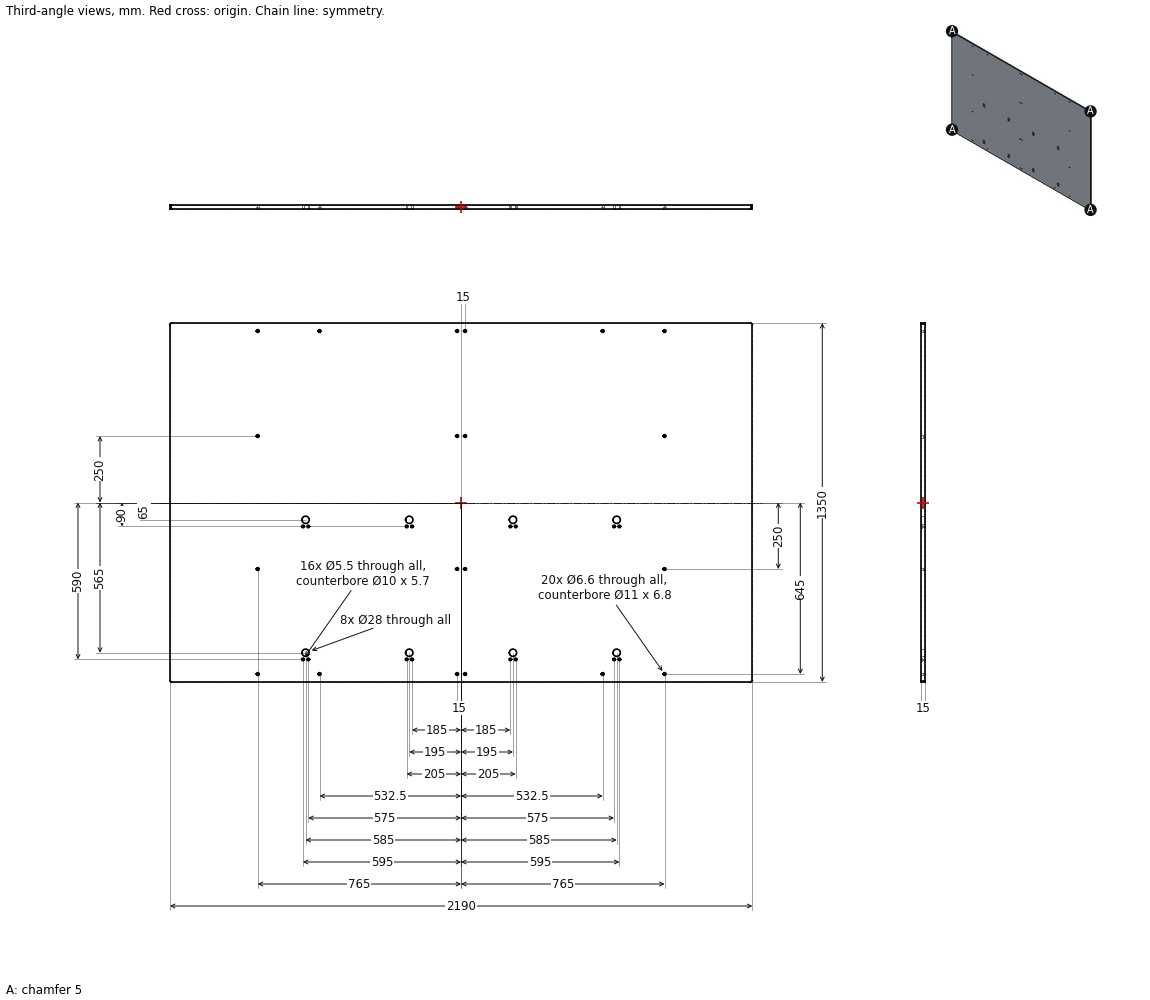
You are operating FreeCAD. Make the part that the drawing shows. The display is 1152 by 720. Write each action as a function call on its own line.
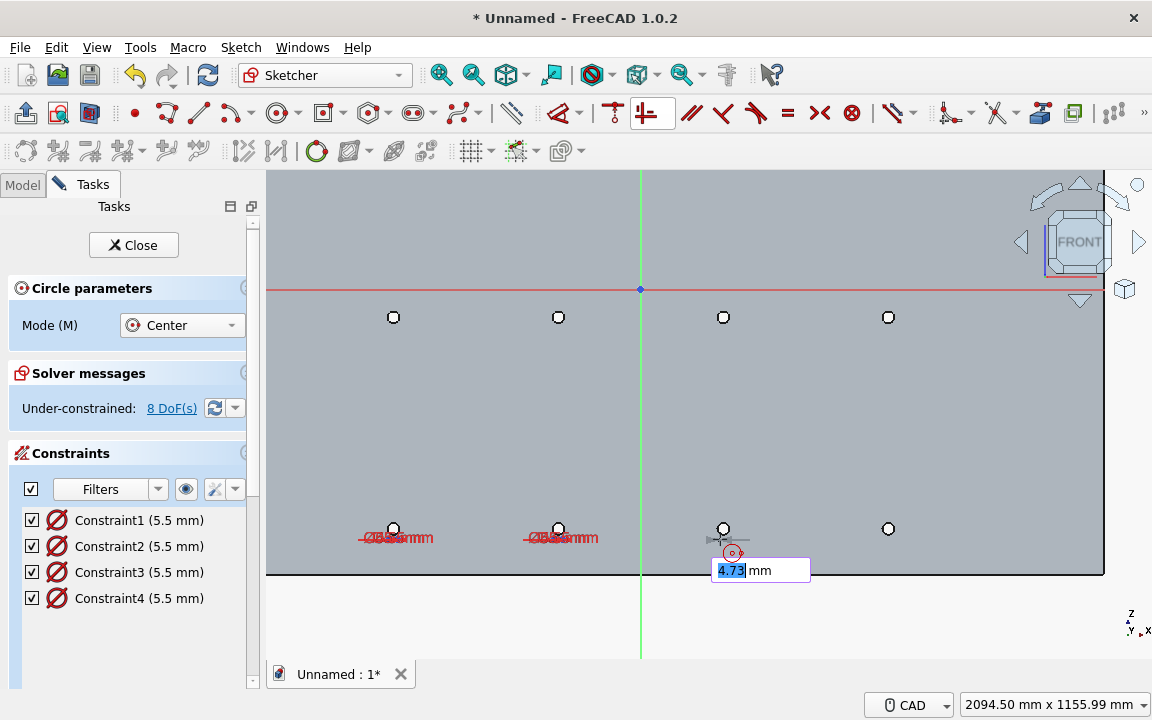
text(5.5)
key(Return)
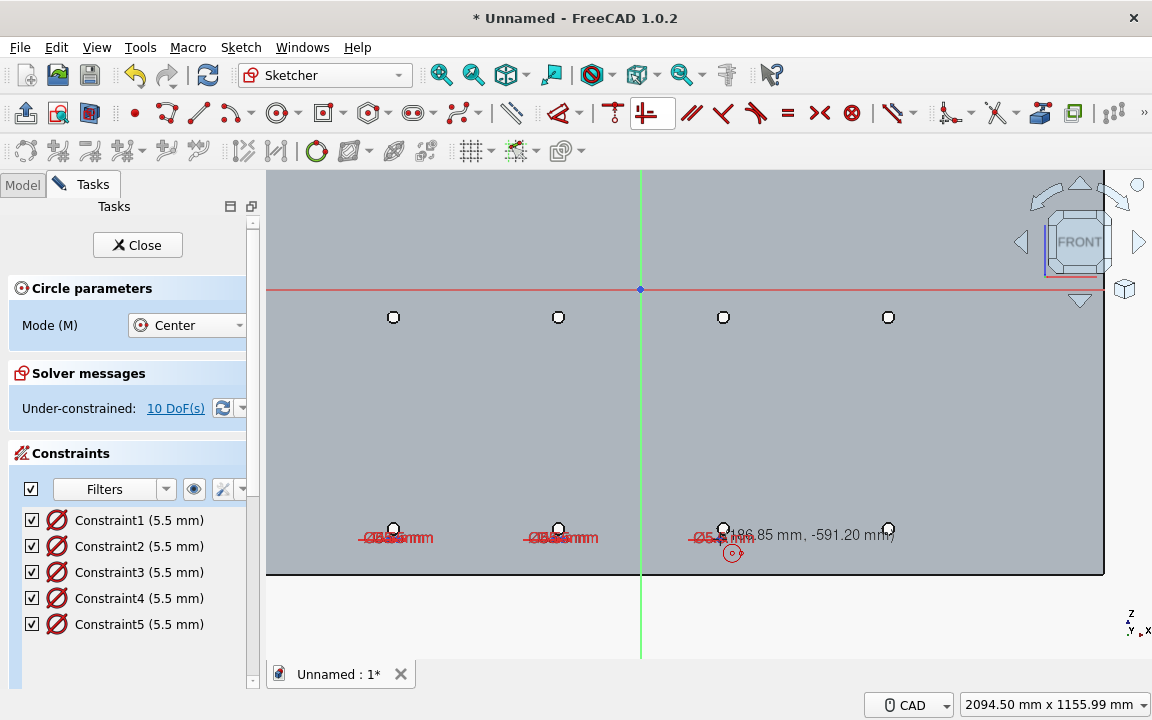
scroll(728, 539, up, 15)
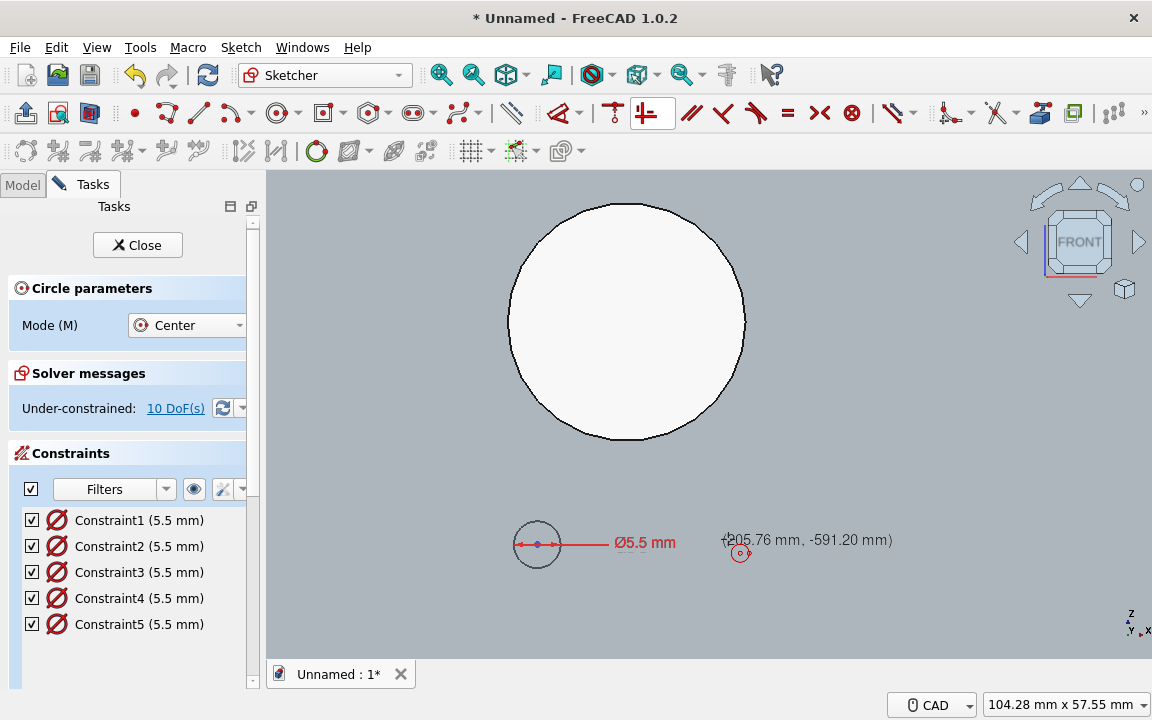
scroll(728, 539, down, 15)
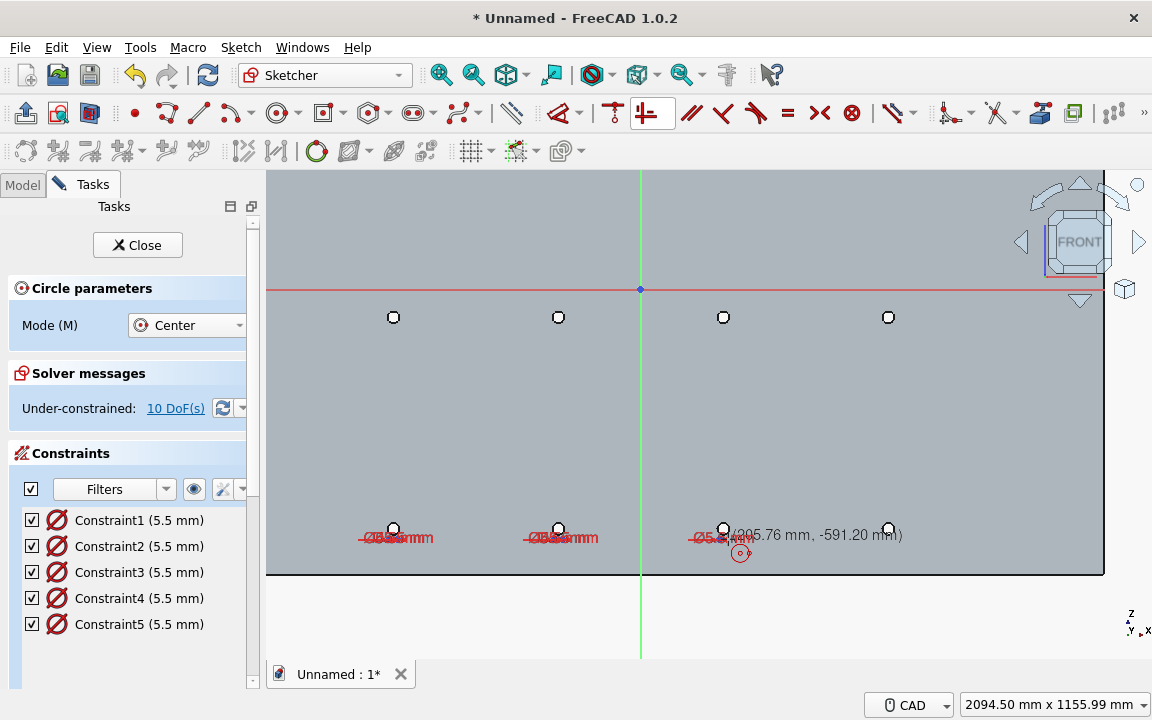
scroll(728, 539, up, 4)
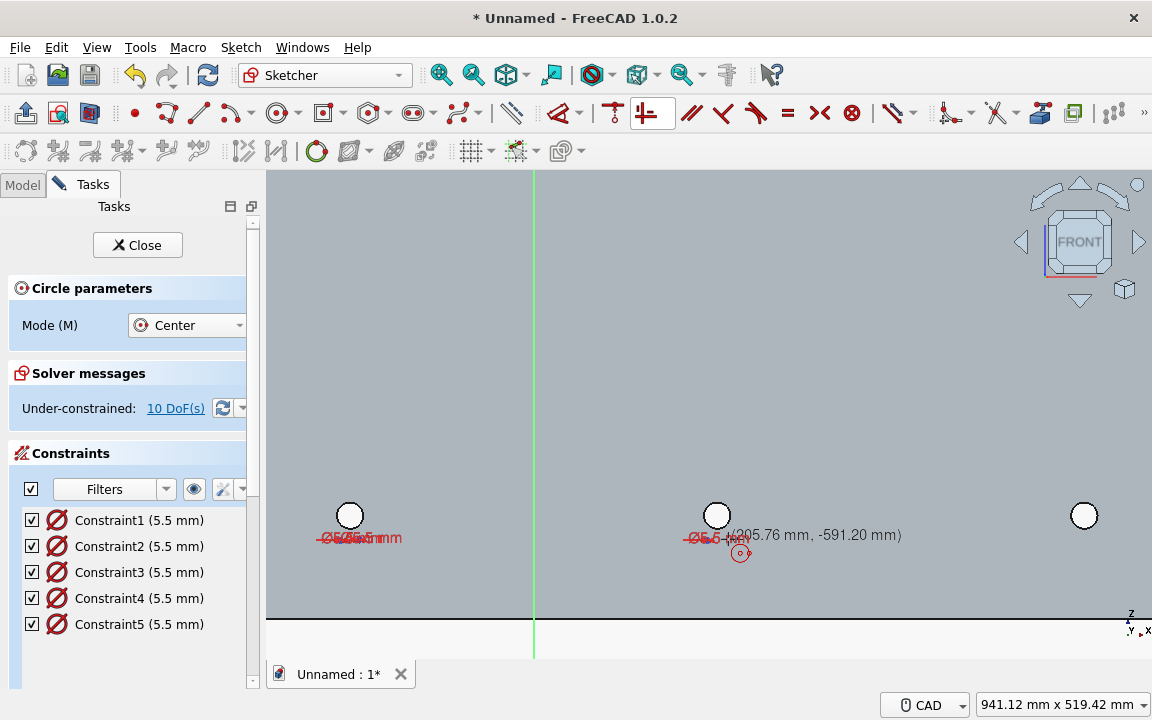
click(727, 539)
move(728, 537)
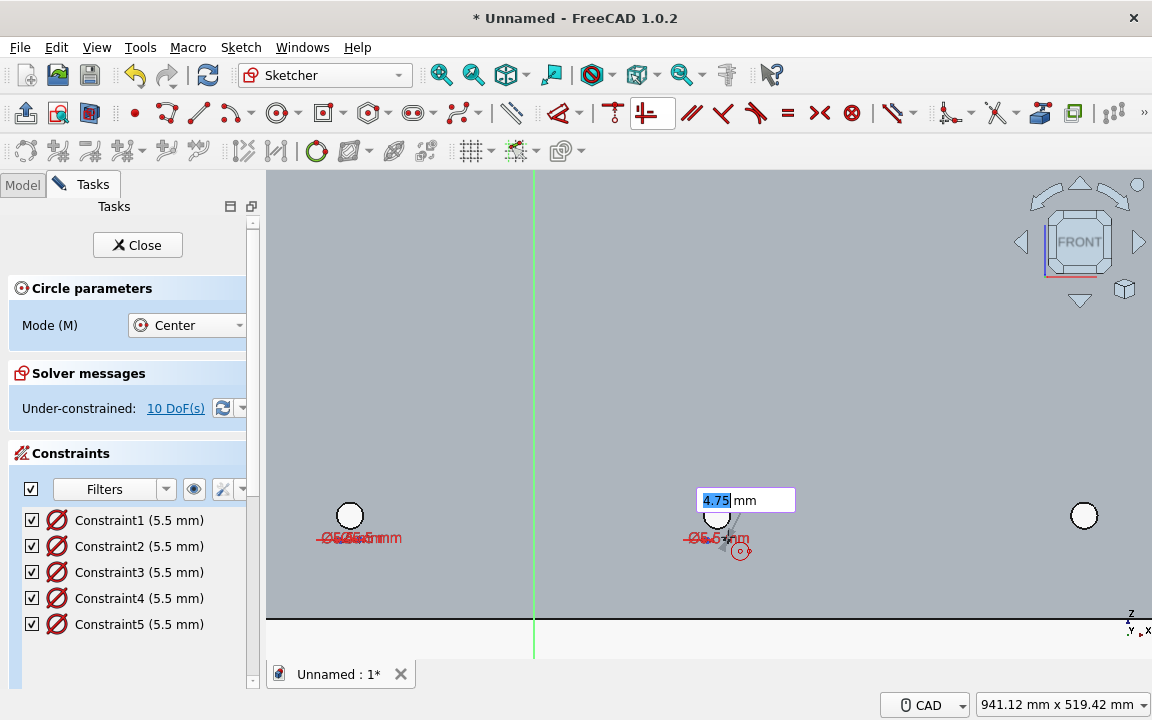
text(5.5)
key(Return)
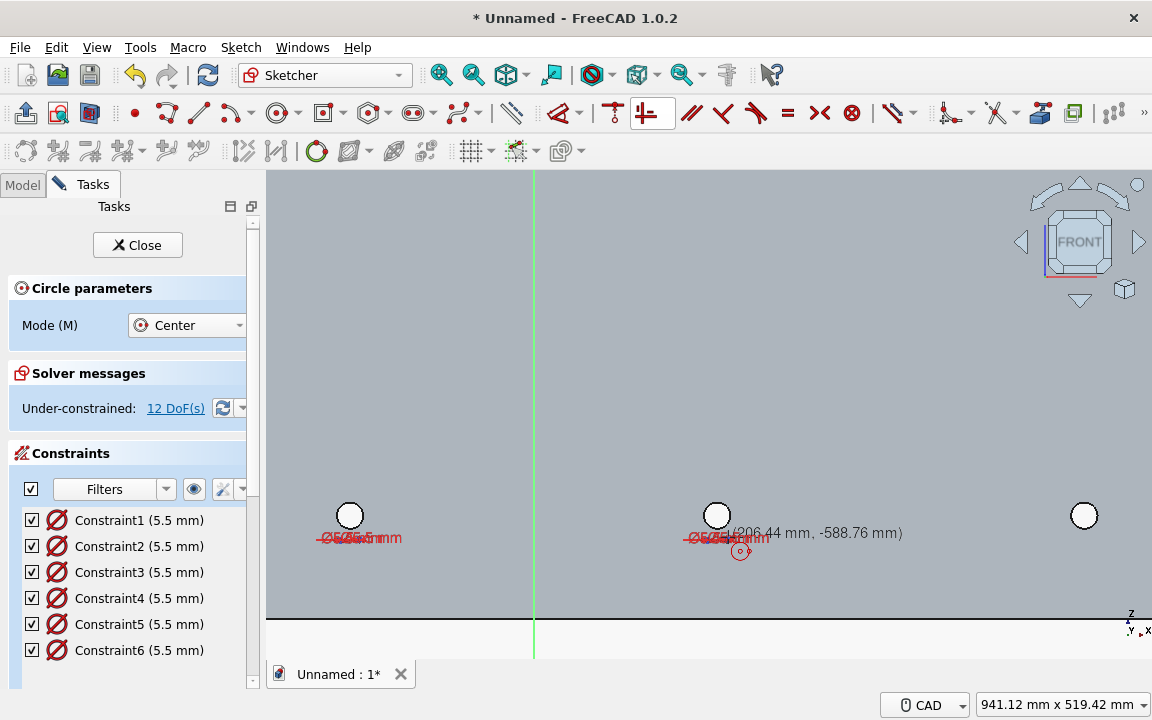
scroll(728, 538, down, 4)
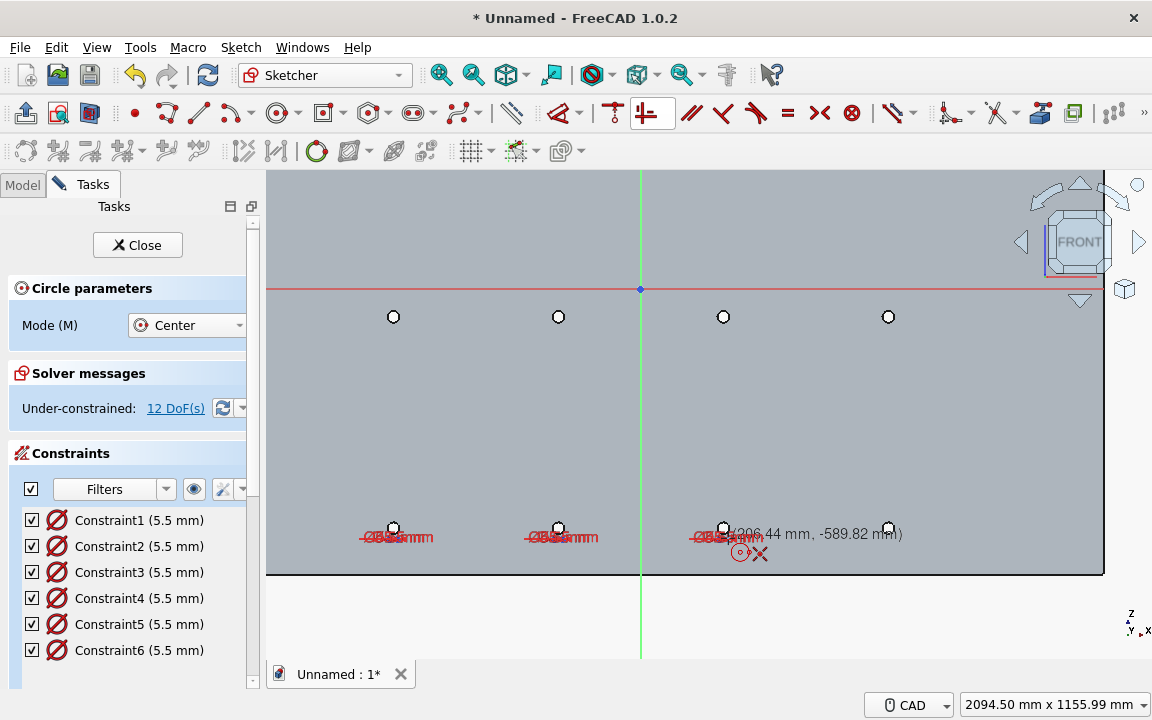
scroll(884, 539, up, 15)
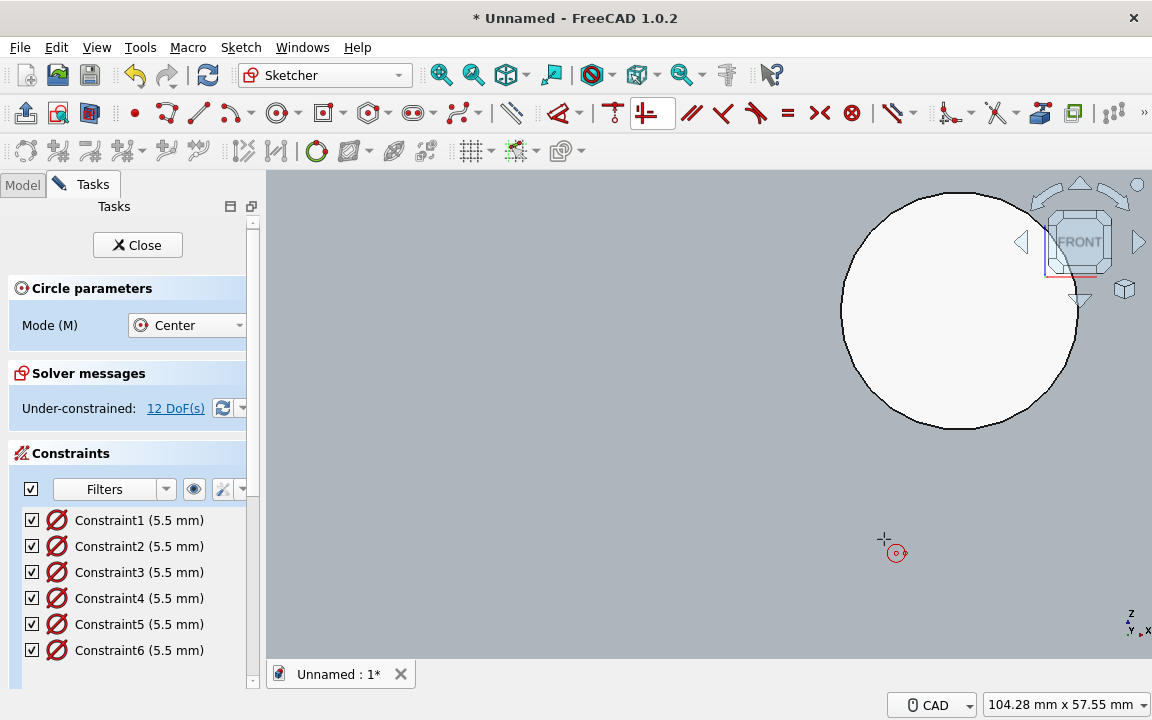
scroll(884, 540, down, 15)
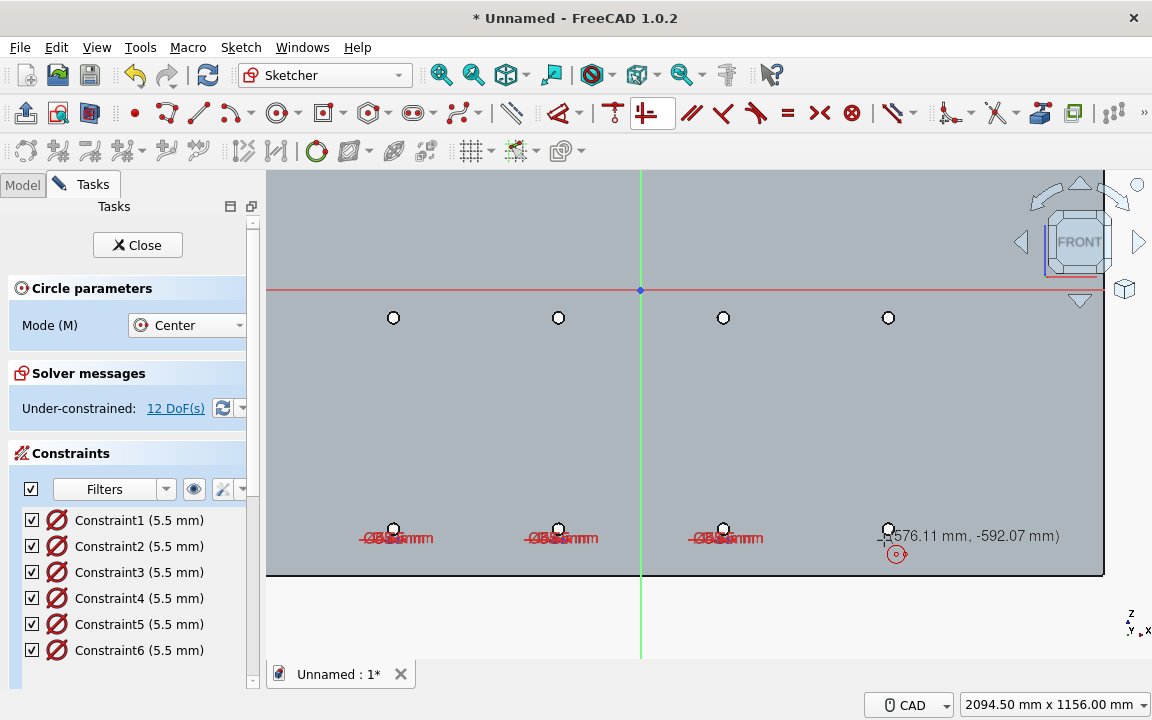
click(884, 540)
move(885, 539)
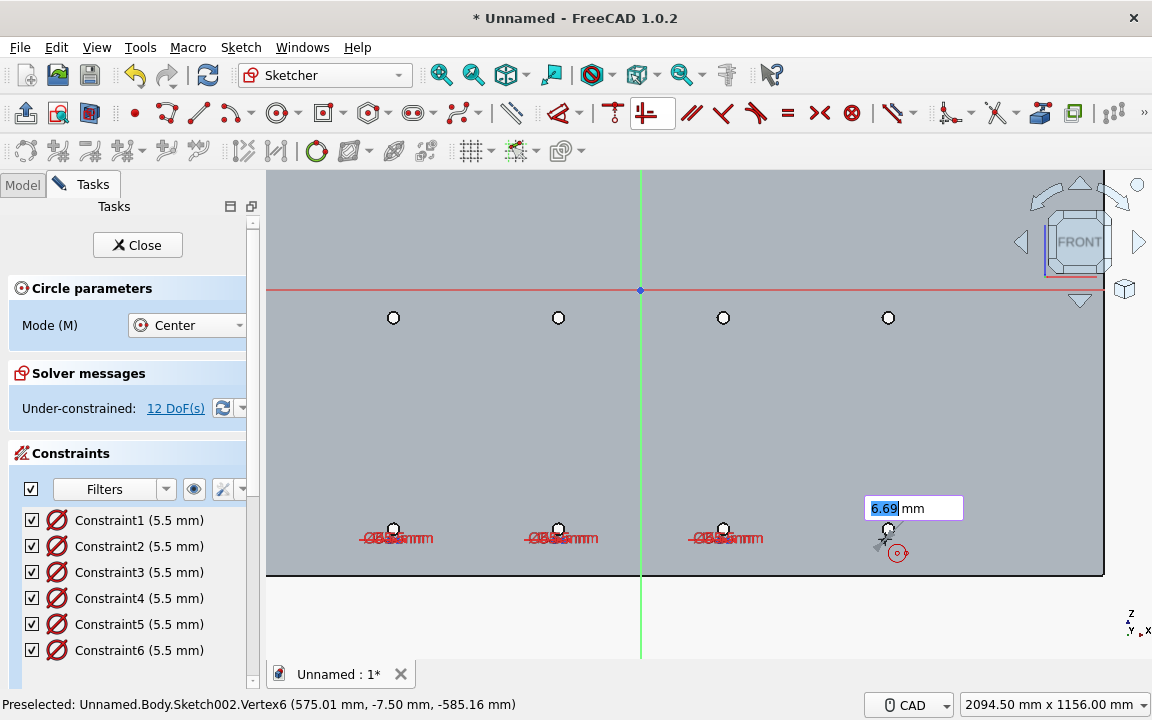
text(5.5)
key(Return)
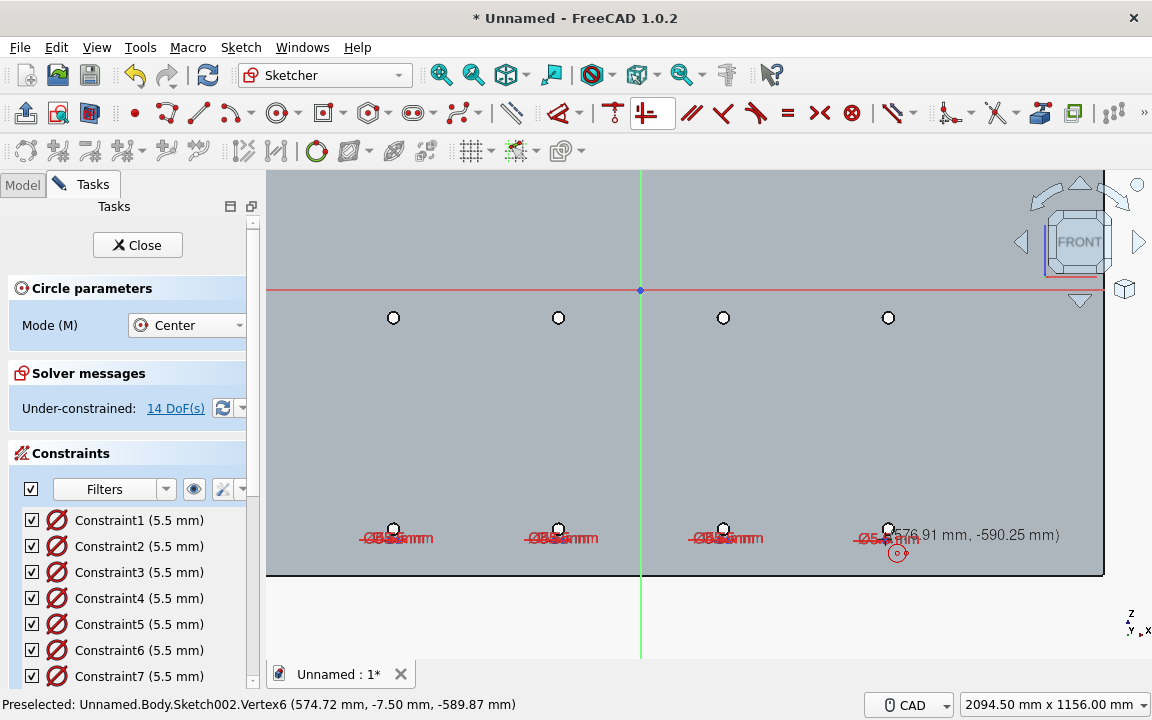
scroll(893, 540, up, 15)